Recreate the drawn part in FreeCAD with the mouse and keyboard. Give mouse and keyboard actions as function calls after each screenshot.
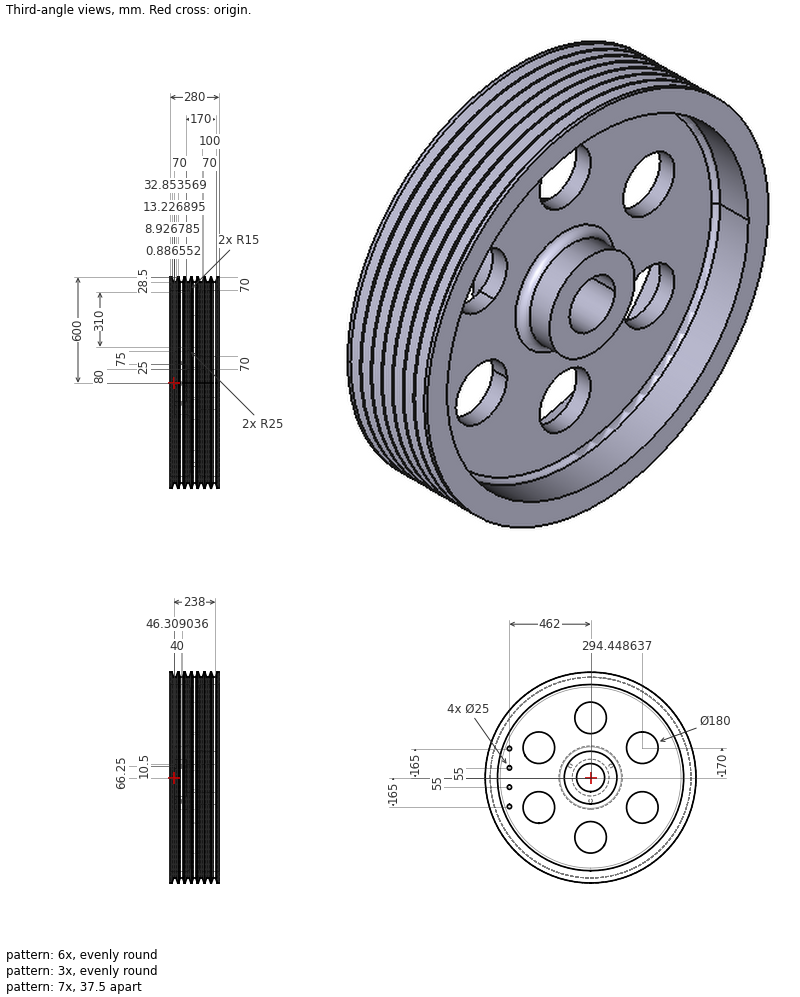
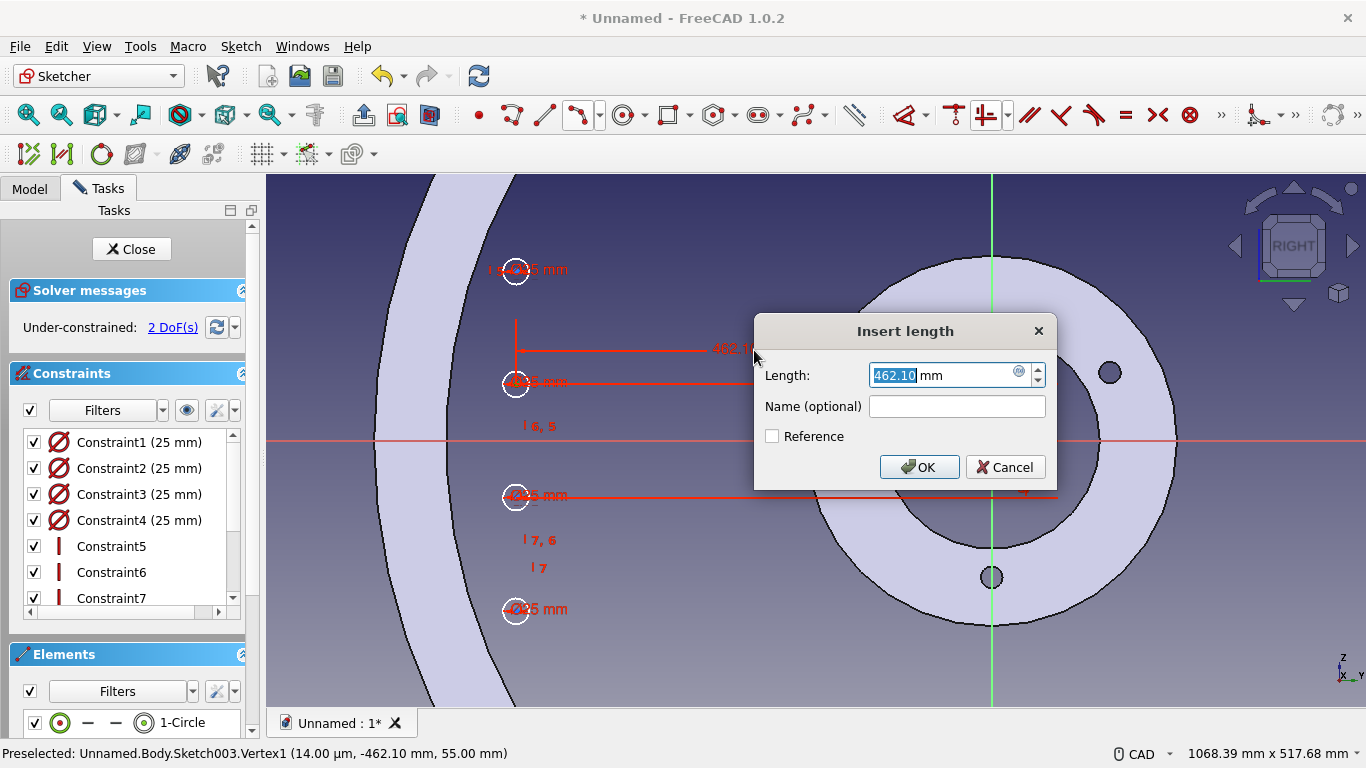
text(462)
key(Return)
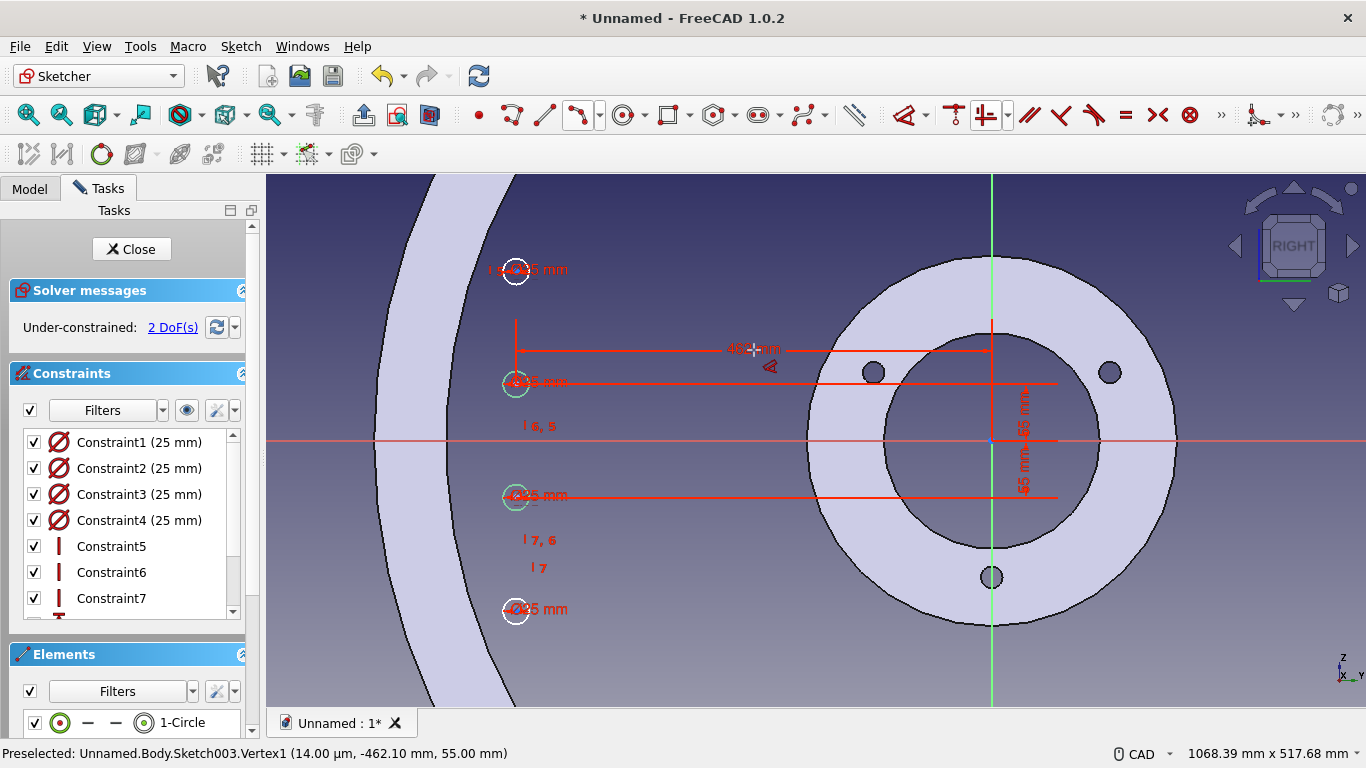
click(516, 272)
click(1026, 356)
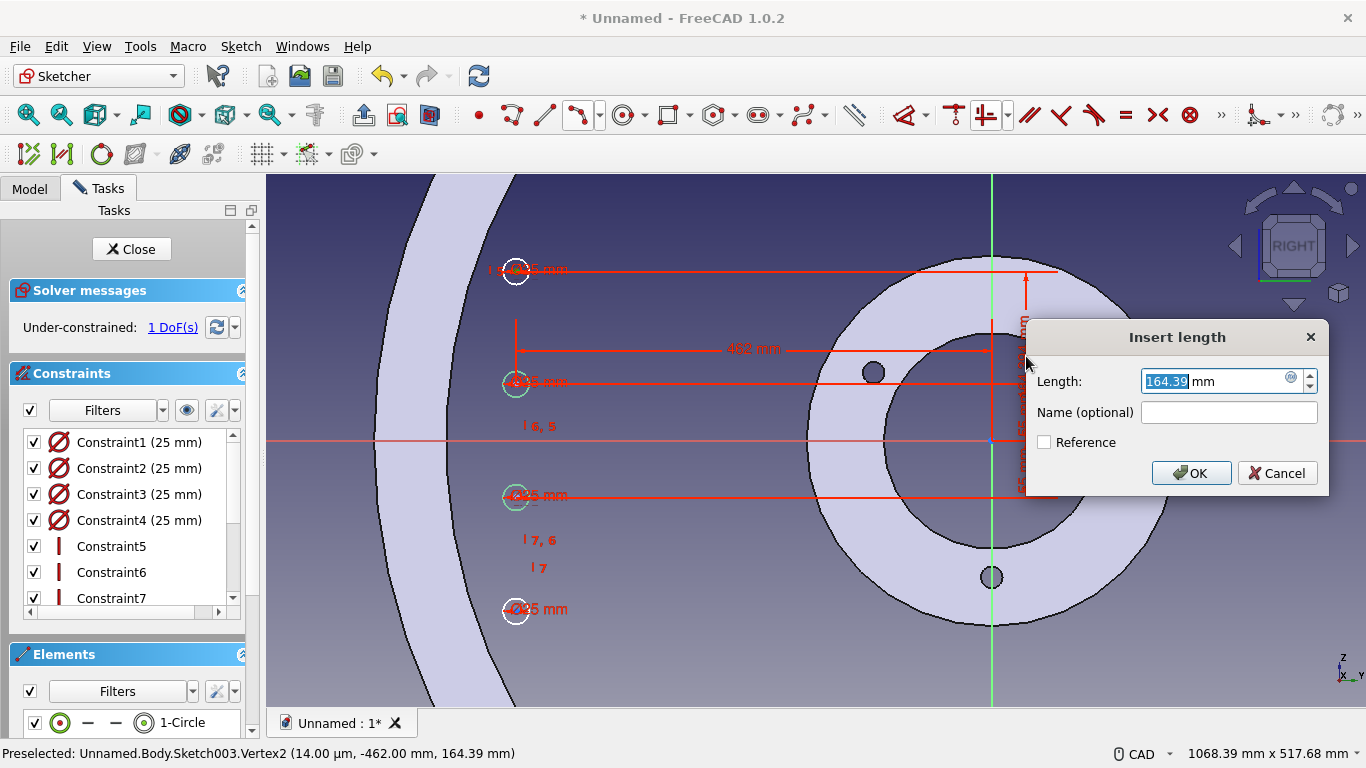
text(165)
key(Return)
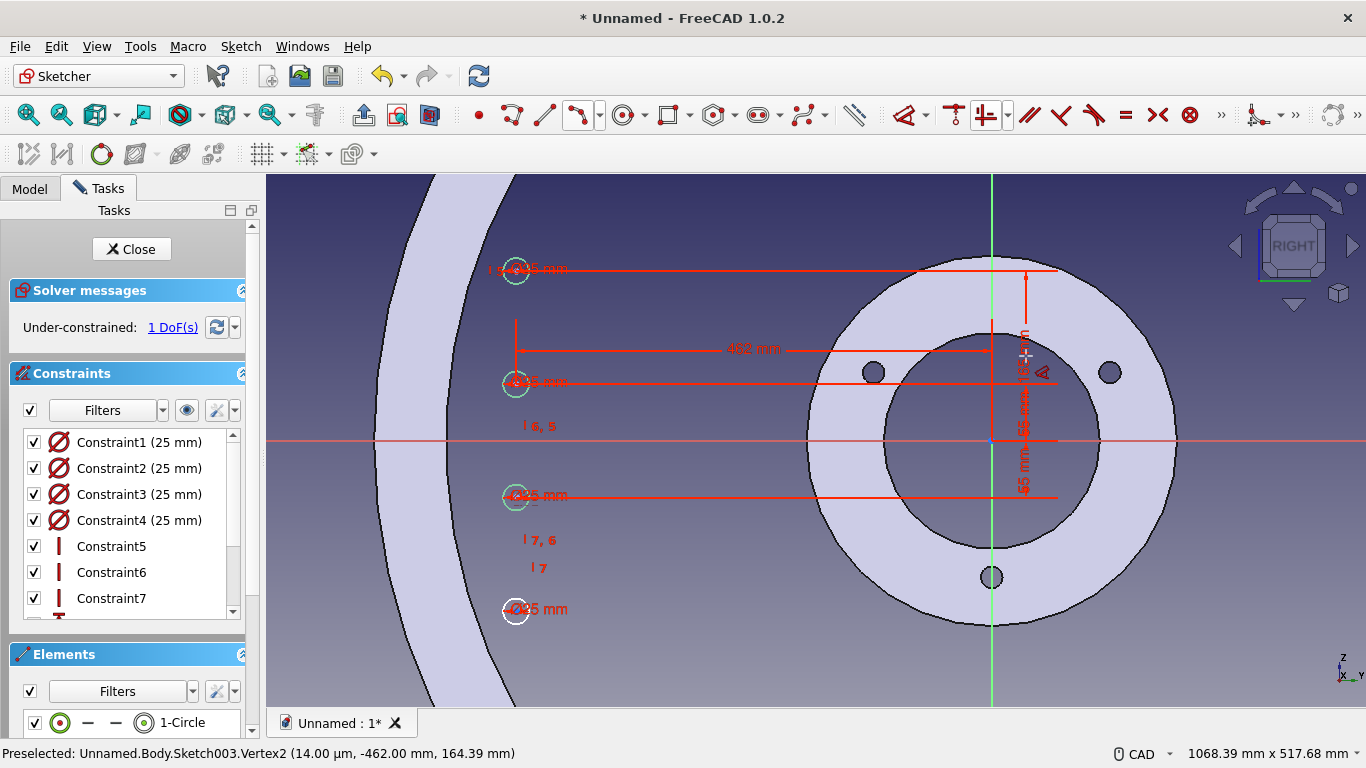
click(516, 611)
click(1026, 526)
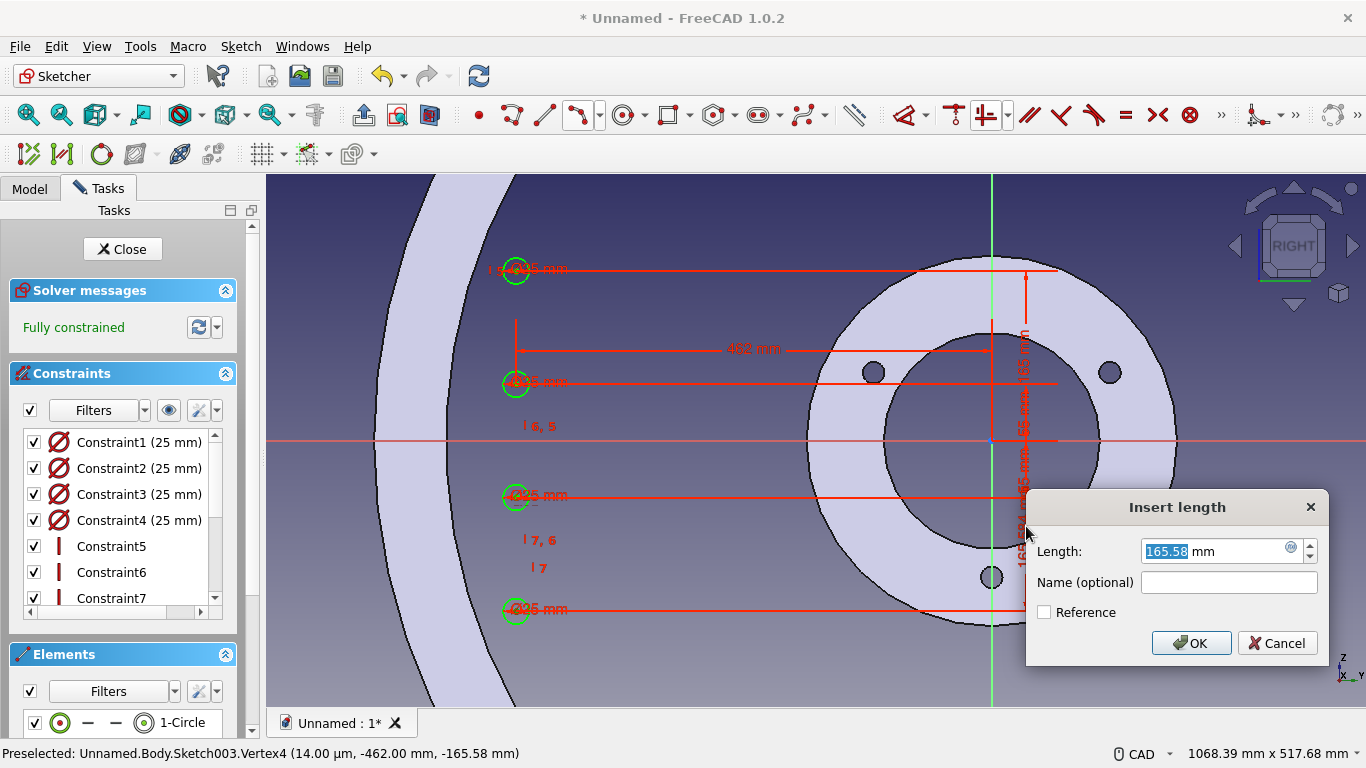
text(165)
key(Return)
key(Escape)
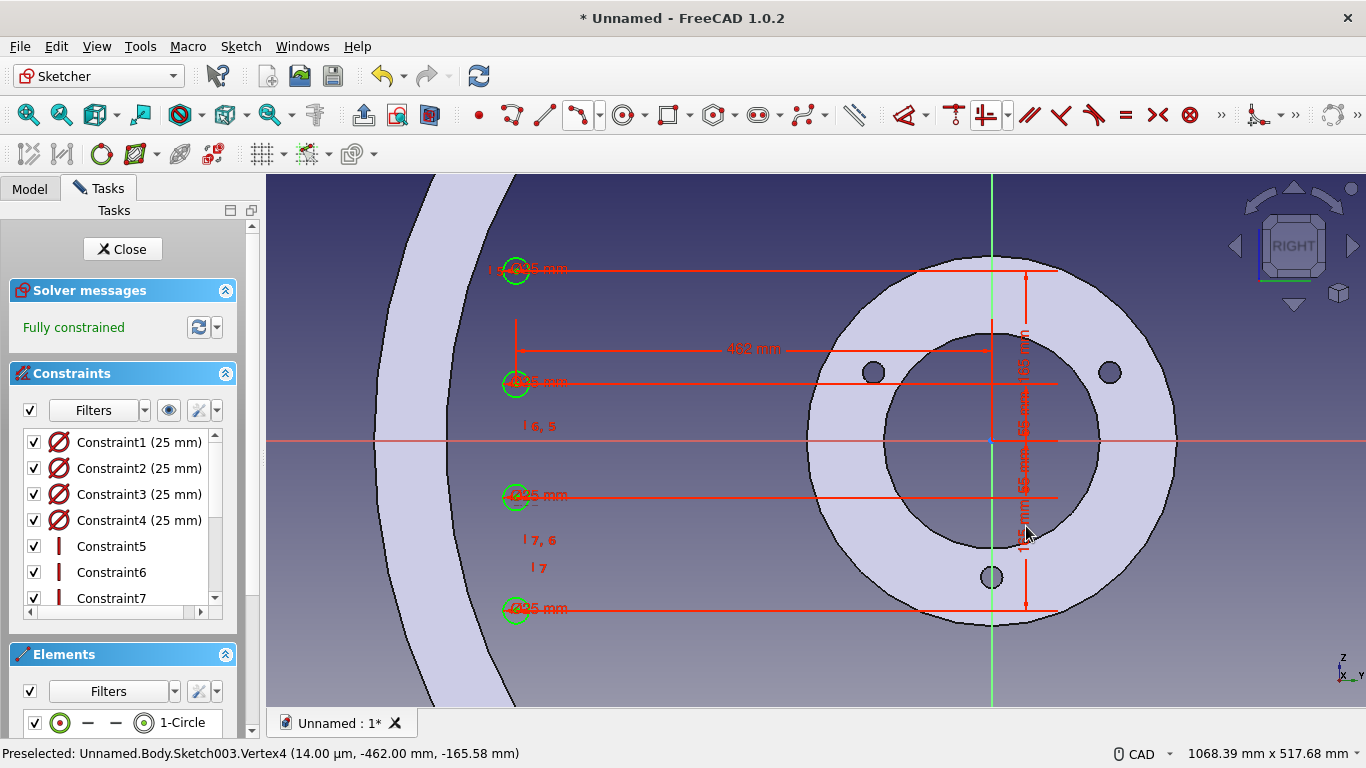
click(123, 249)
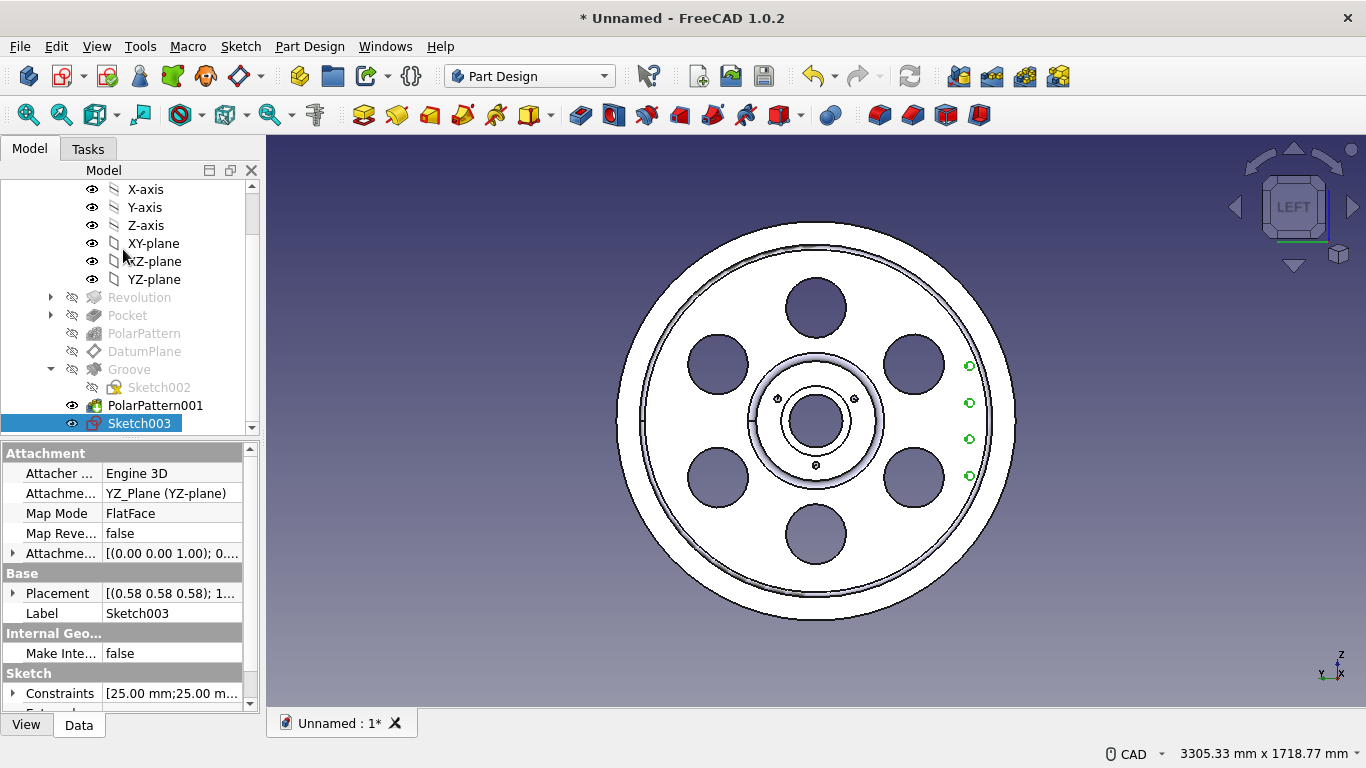
click(581, 116)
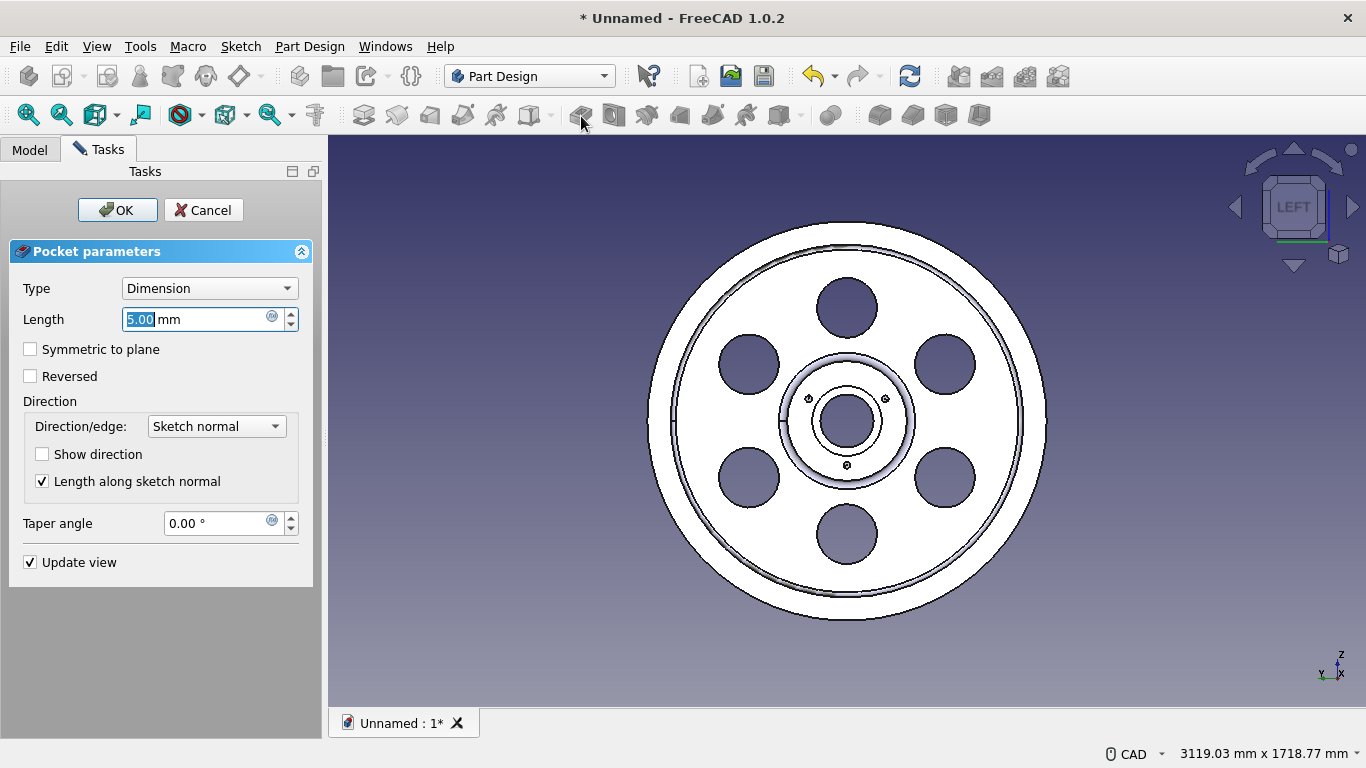
text(238)
key(Tab)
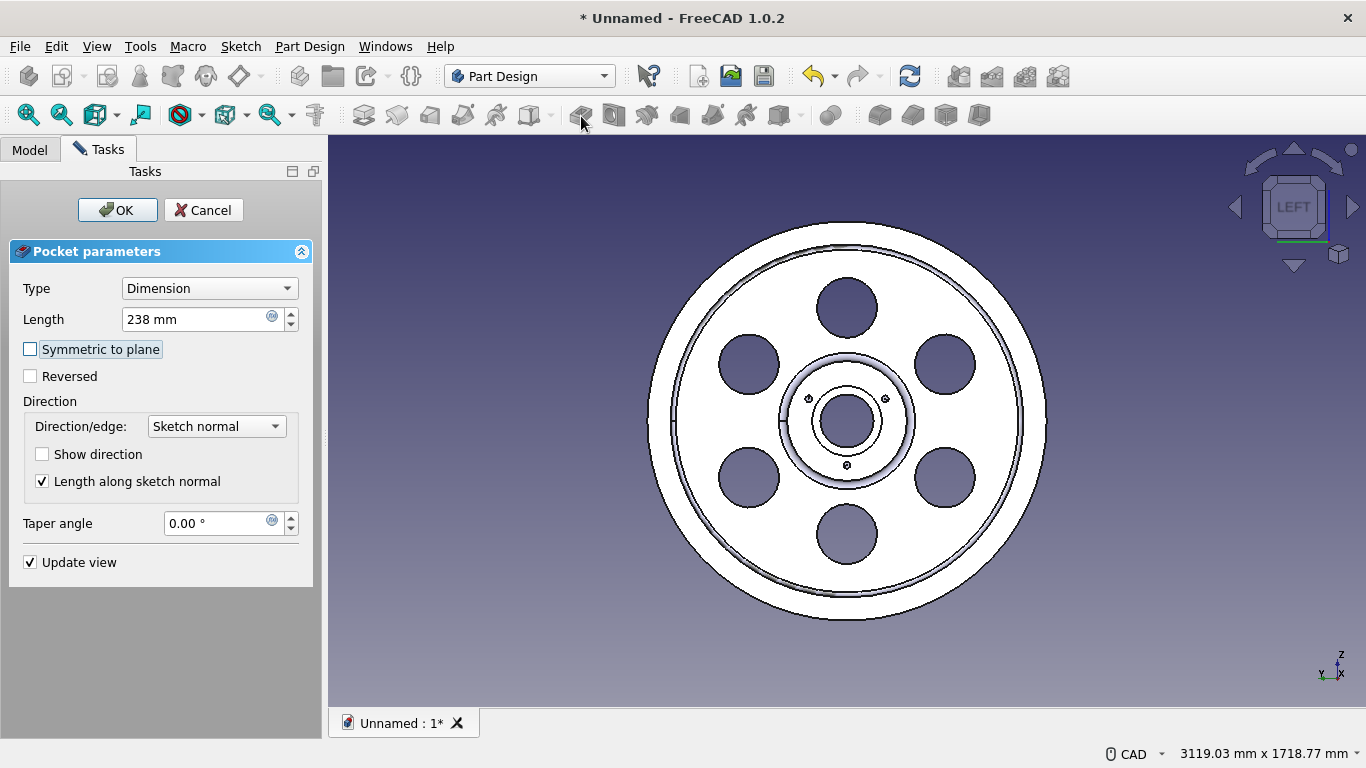
click(31, 376)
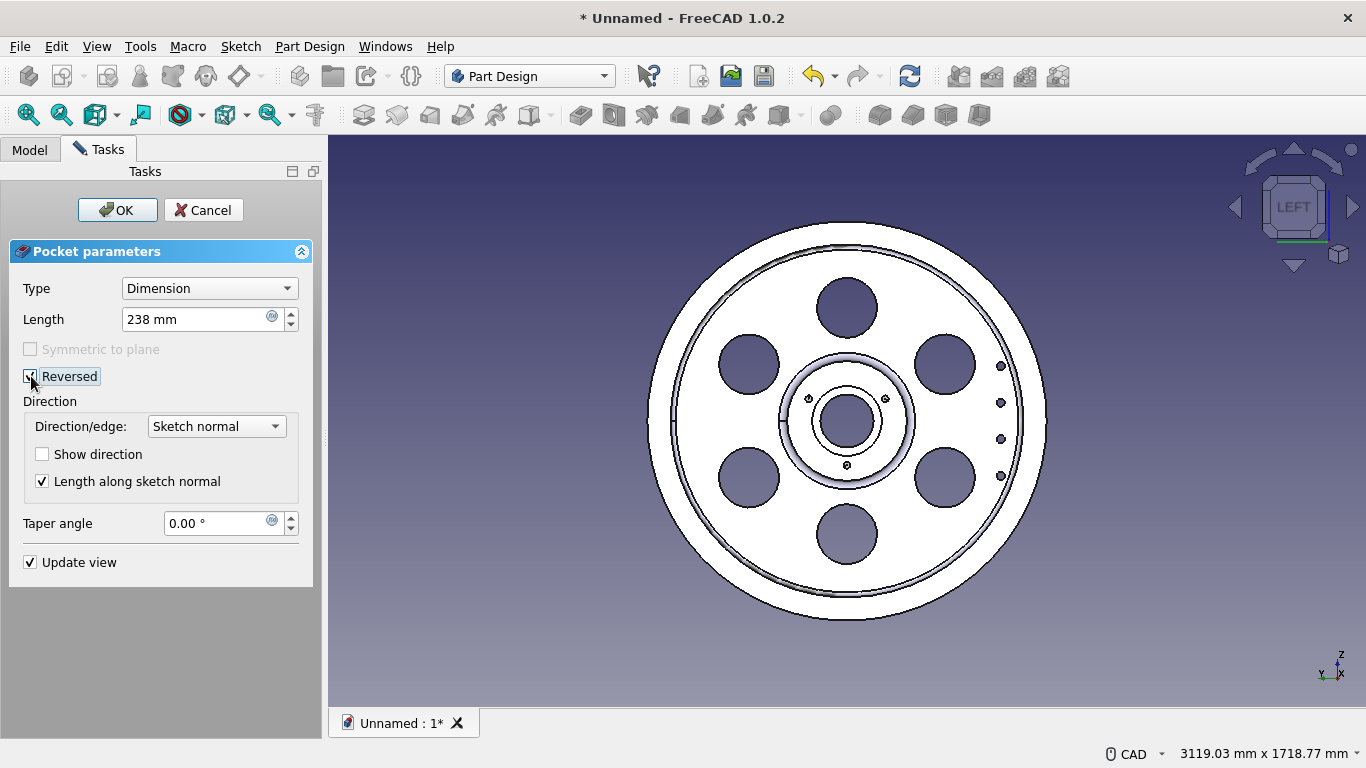
click(118, 210)